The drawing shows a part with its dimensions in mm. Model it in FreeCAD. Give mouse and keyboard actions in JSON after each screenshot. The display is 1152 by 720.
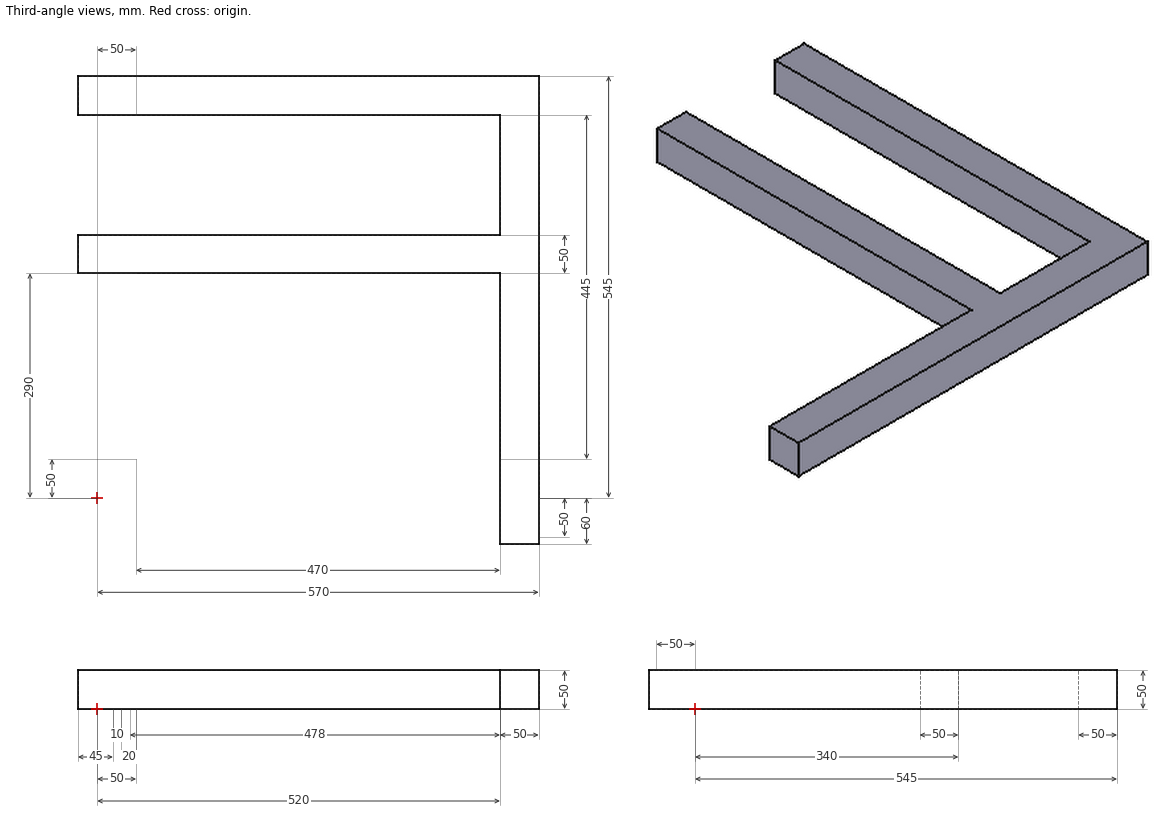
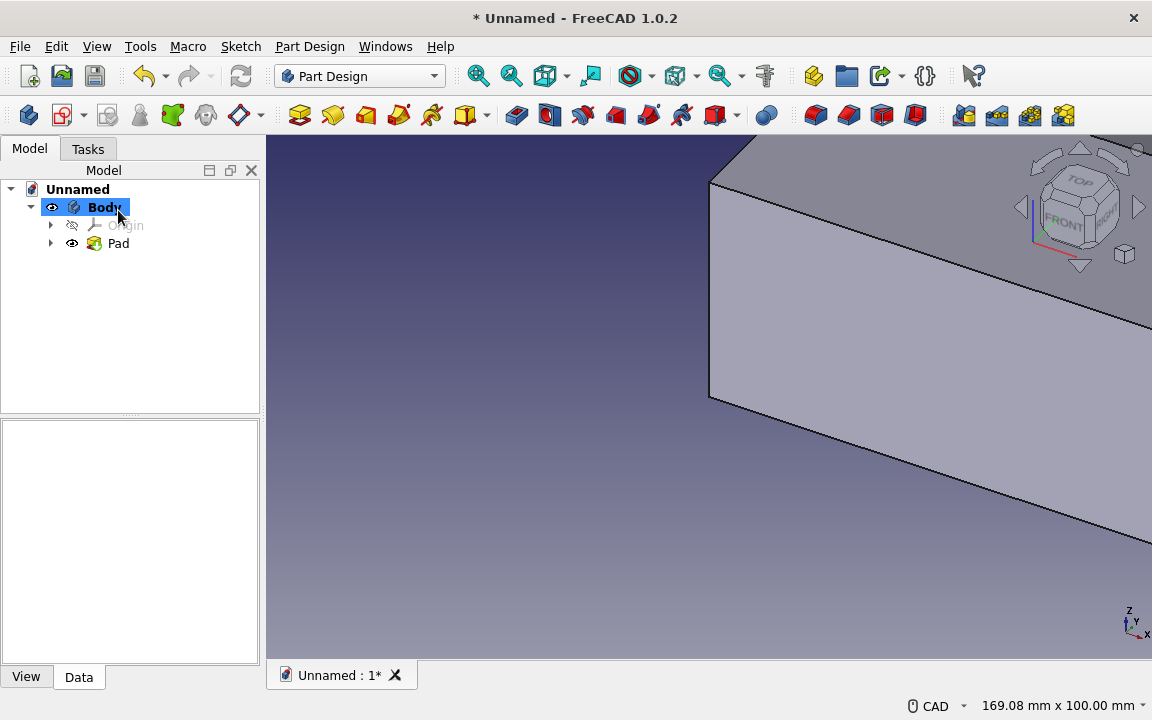
{"action": "left_click", "coordinate": [479, 76]}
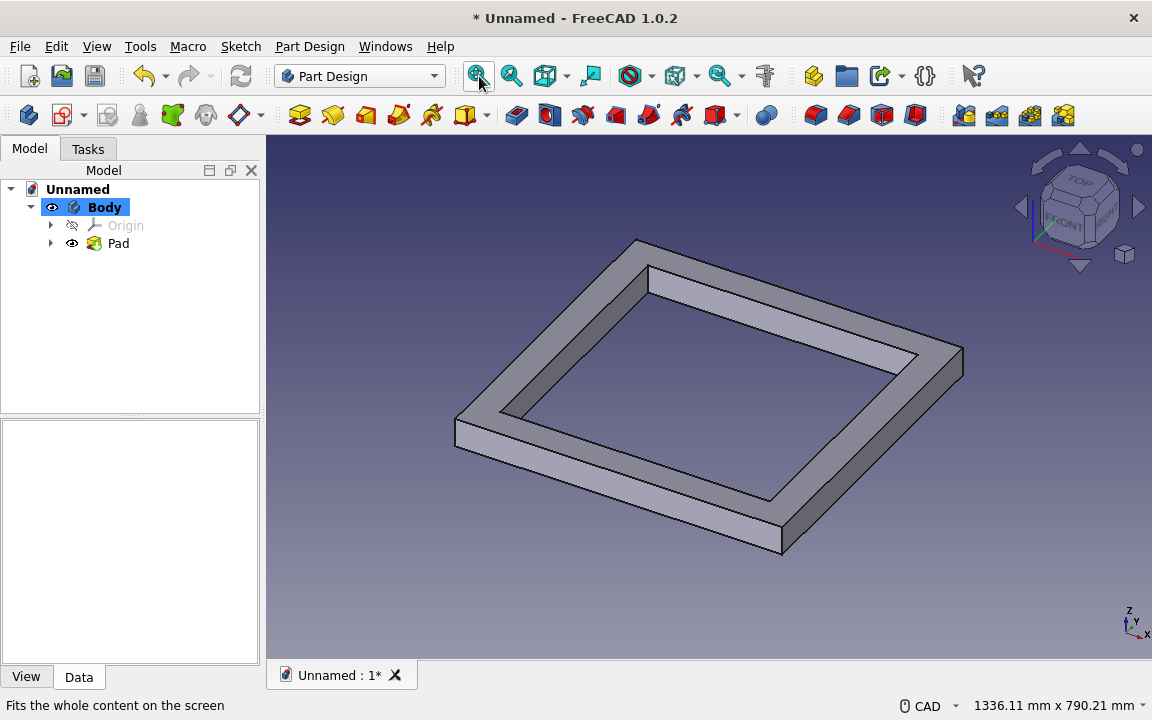
{"action": "key", "text": "5"}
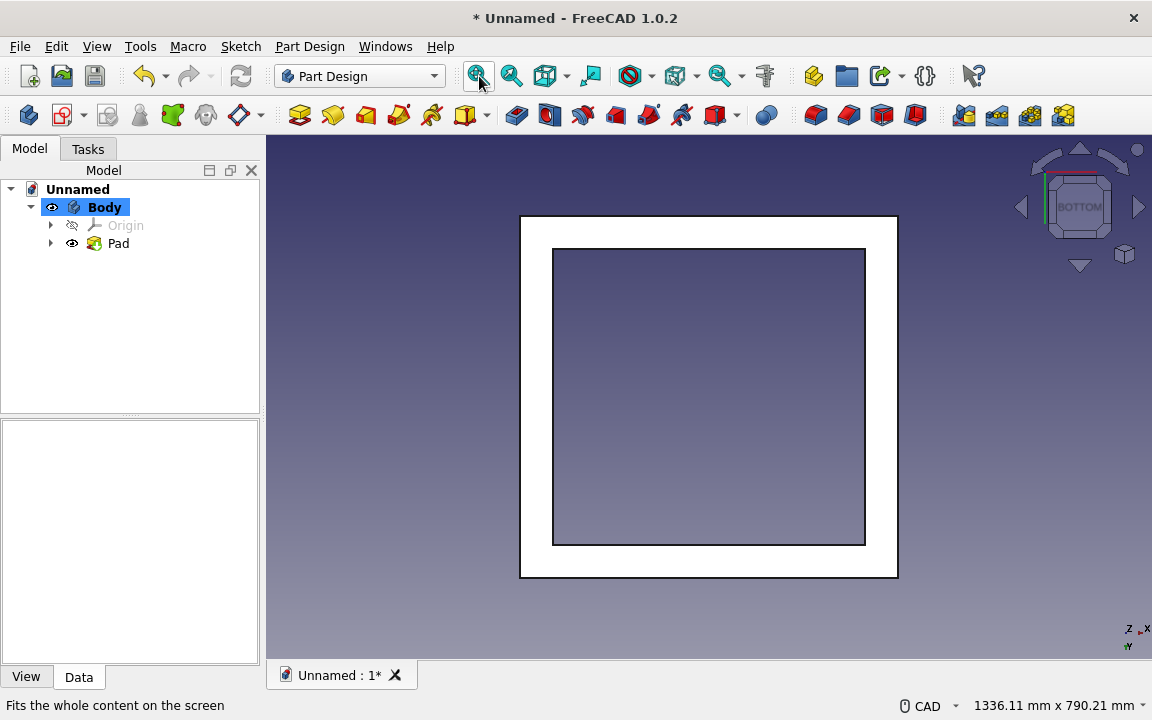
{"action": "left_click", "coordinate": [871, 551]}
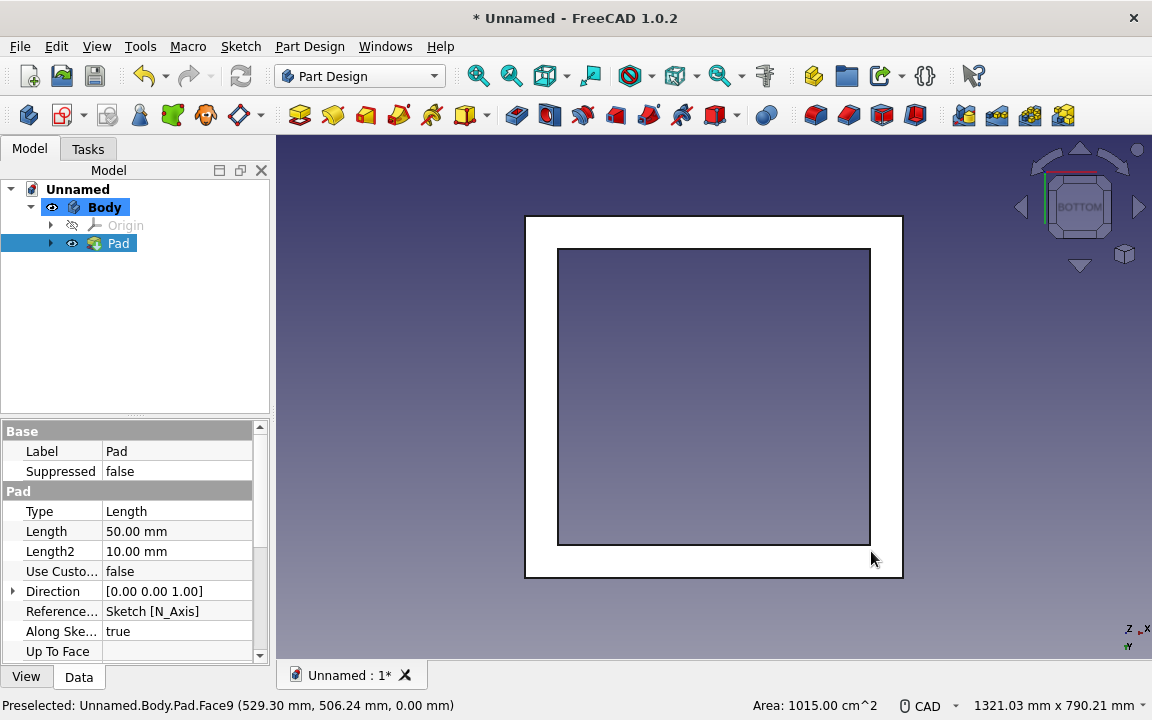
{"action": "left_click", "coordinate": [62, 116]}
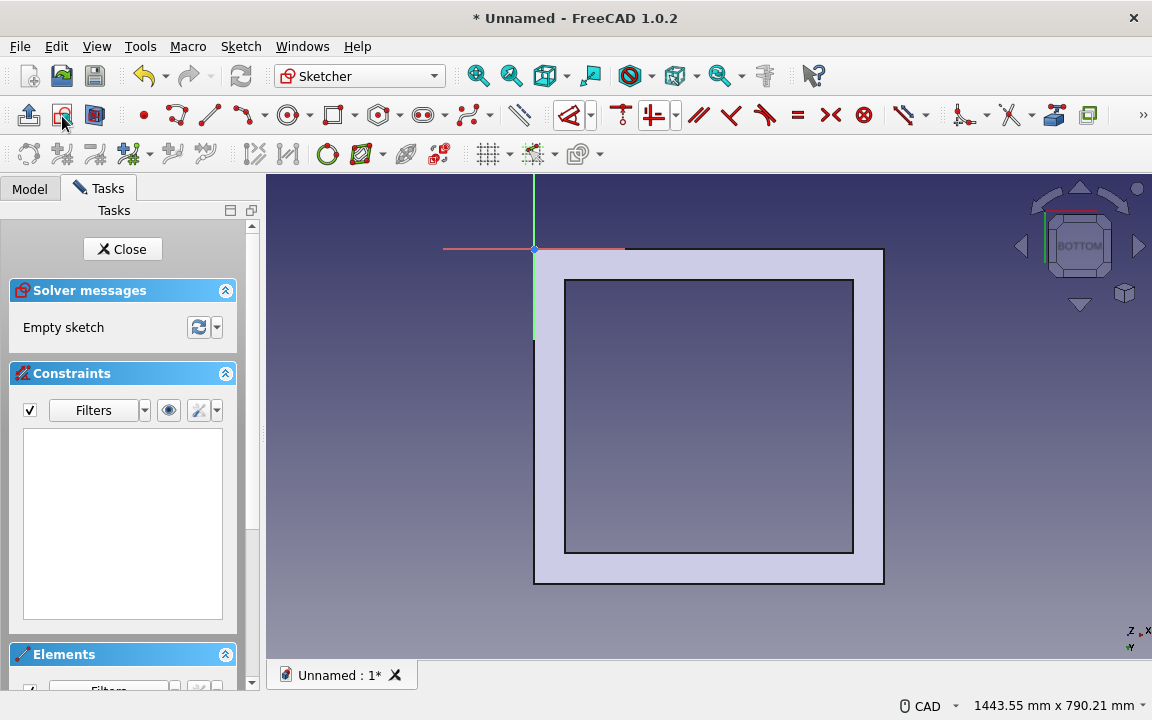
{"action": "scroll", "coordinate": [802, 226], "scroll_direction": "up", "scroll_amount": 2}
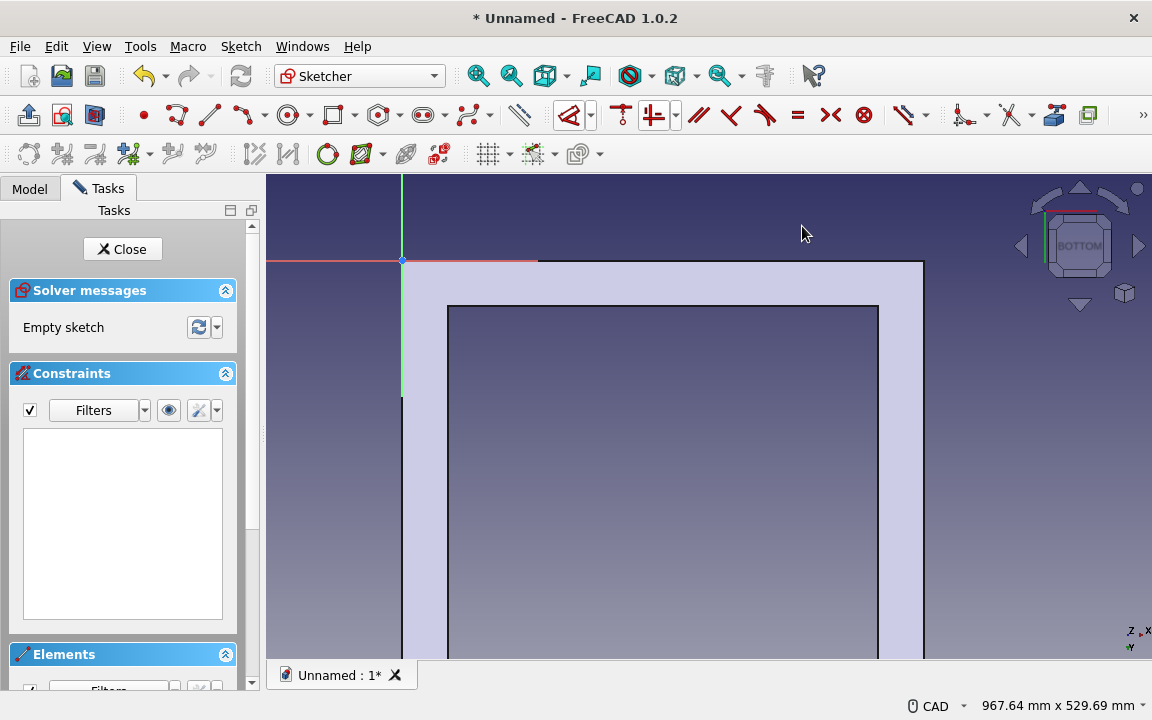
{"action": "left_click", "coordinate": [332, 116]}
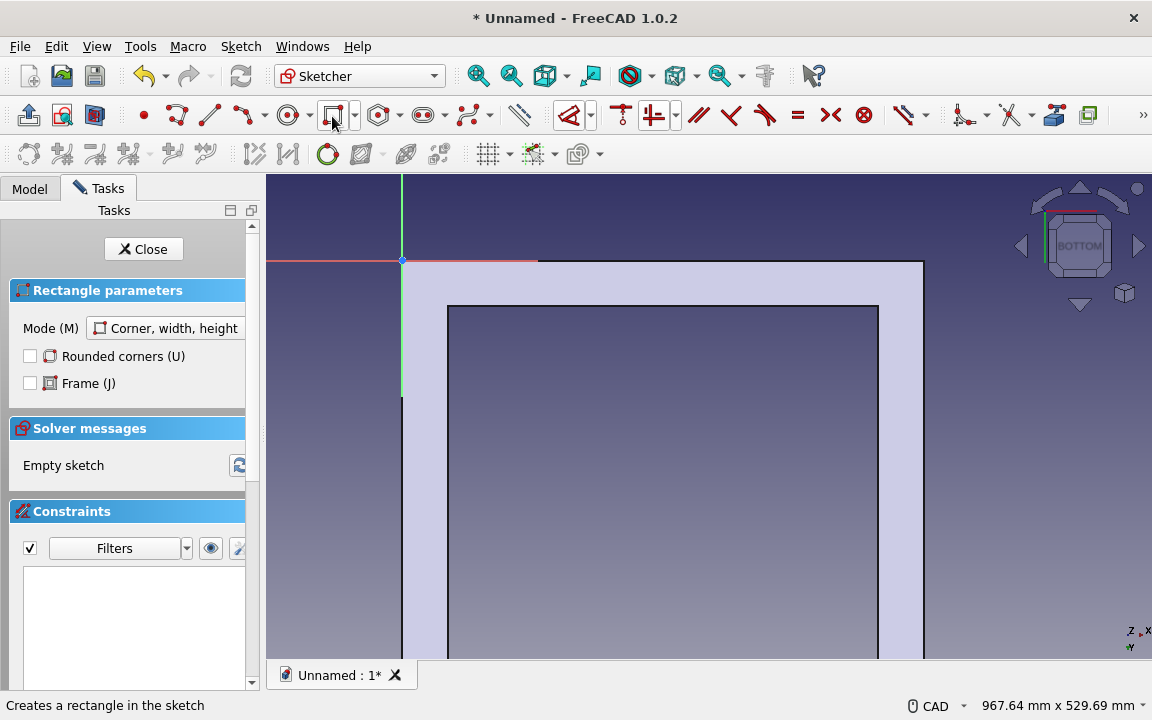
{"action": "left_click", "coordinate": [448, 526]}
{"action": "mouse_move", "coordinate": [878, 572]}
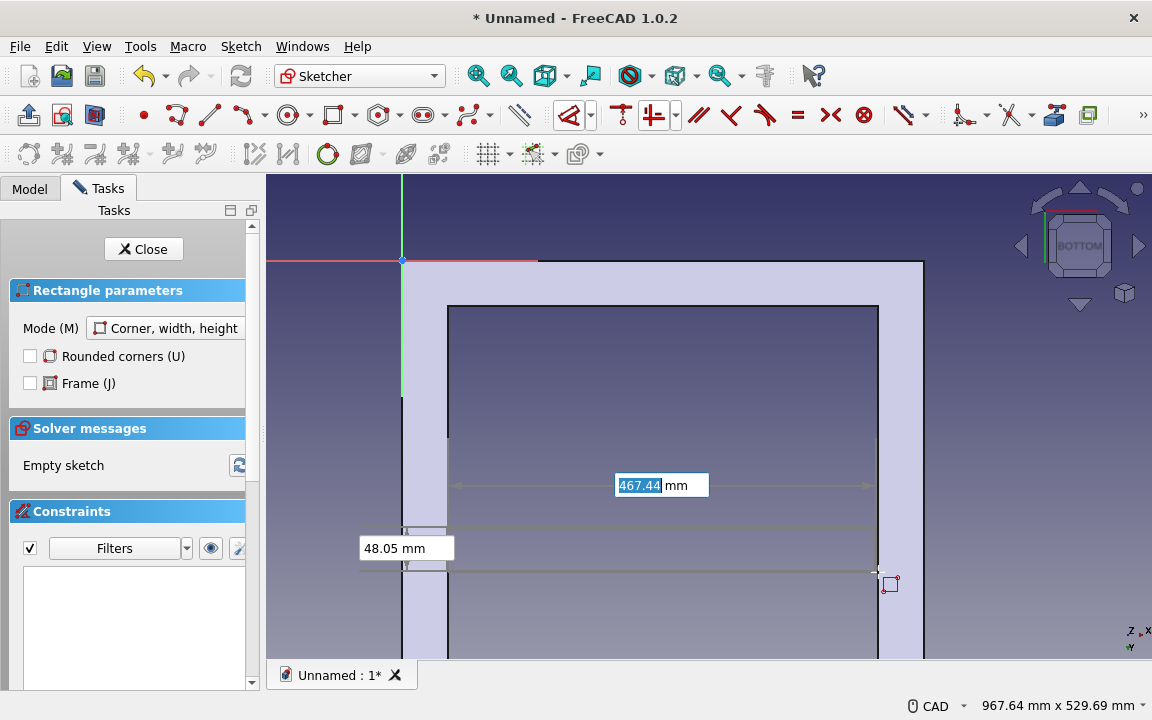
{"action": "type", "text": "470"}
{"action": "key", "text": "Tab"}
{"action": "type", "text": "50"}
{"action": "key", "text": "Return"}
{"action": "key", "text": "Escape"}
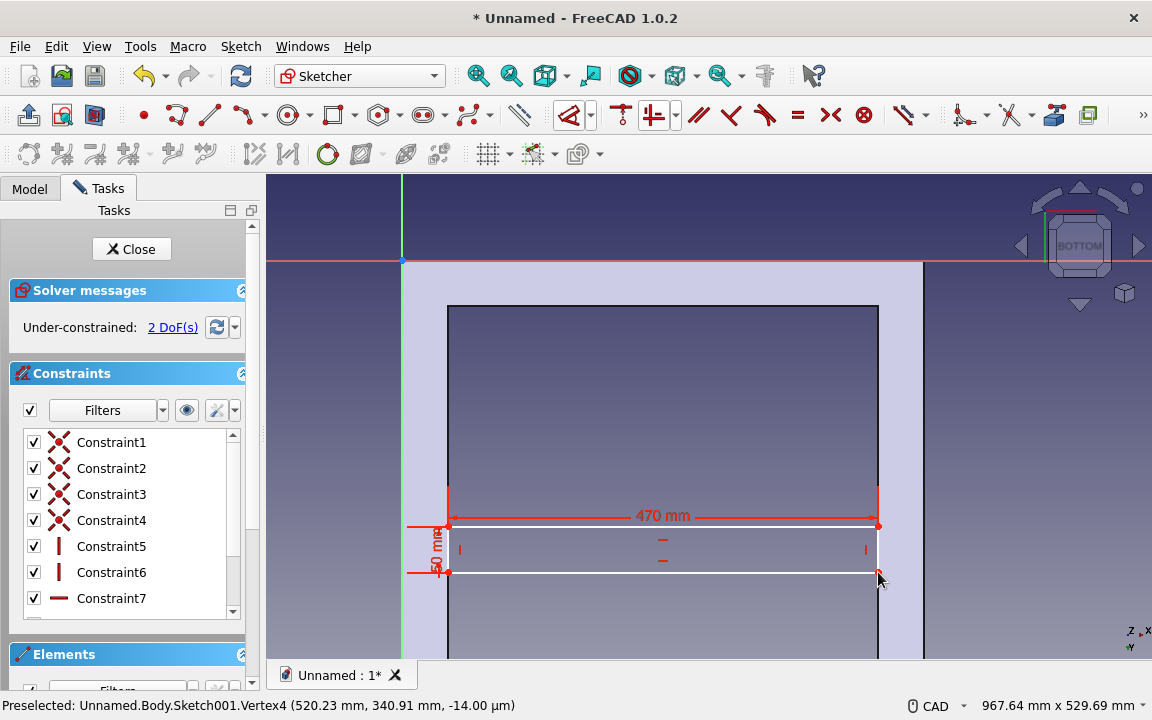
{"action": "left_click", "coordinate": [448, 527]}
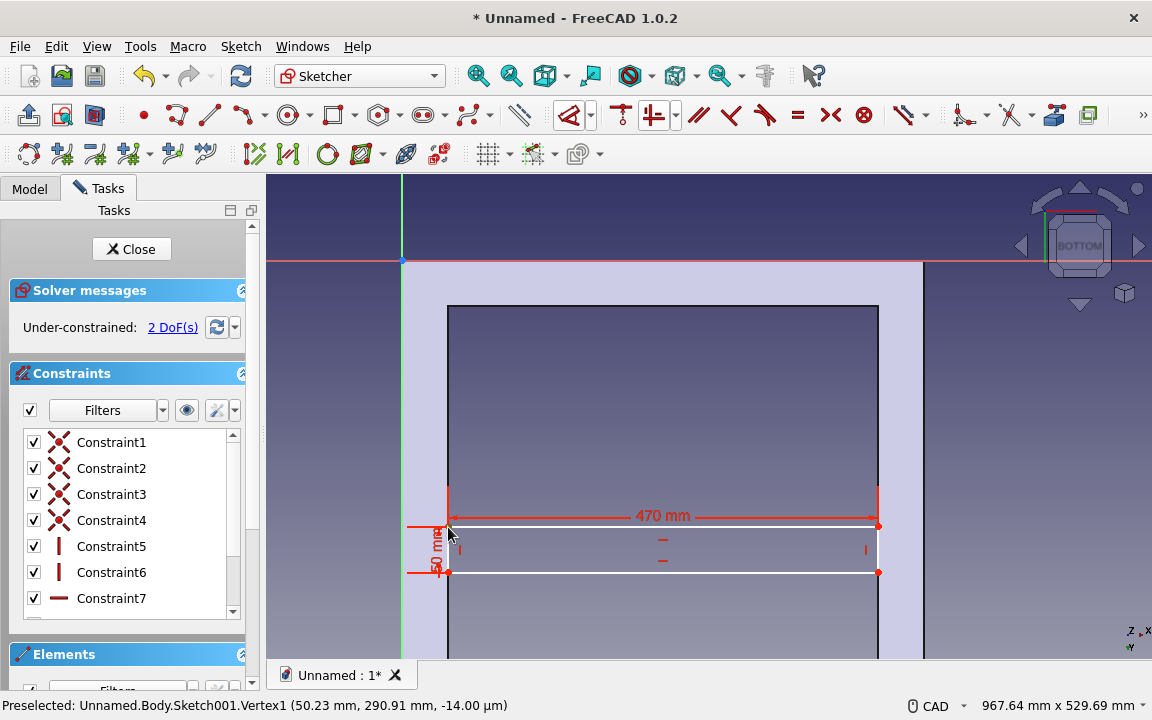
{"action": "left_click", "coordinate": [590, 116]}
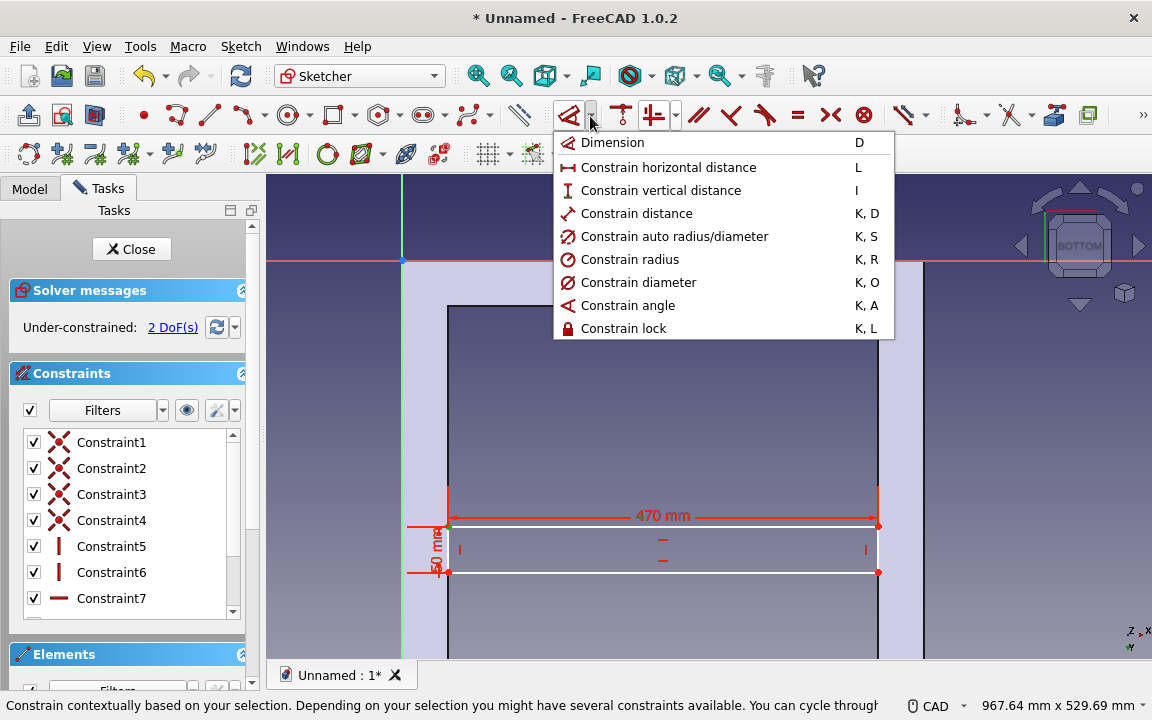
{"action": "left_click", "coordinate": [724, 168]}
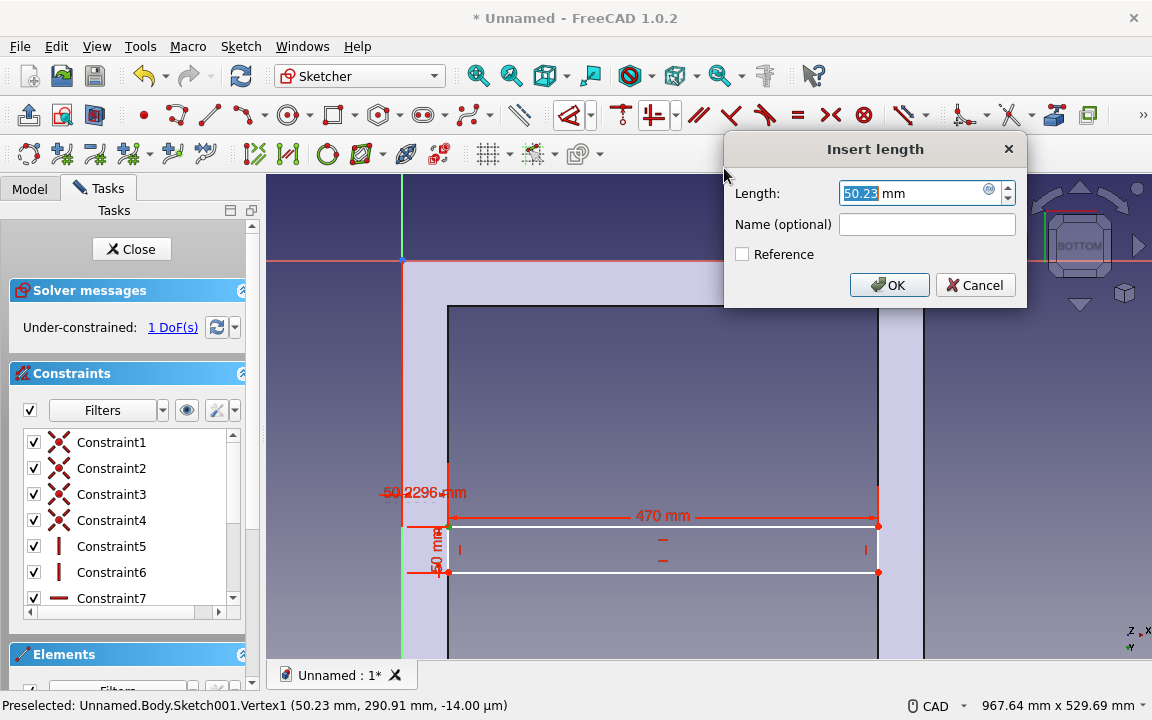
{"action": "type", "text": "50"}
{"action": "key", "text": "Return"}